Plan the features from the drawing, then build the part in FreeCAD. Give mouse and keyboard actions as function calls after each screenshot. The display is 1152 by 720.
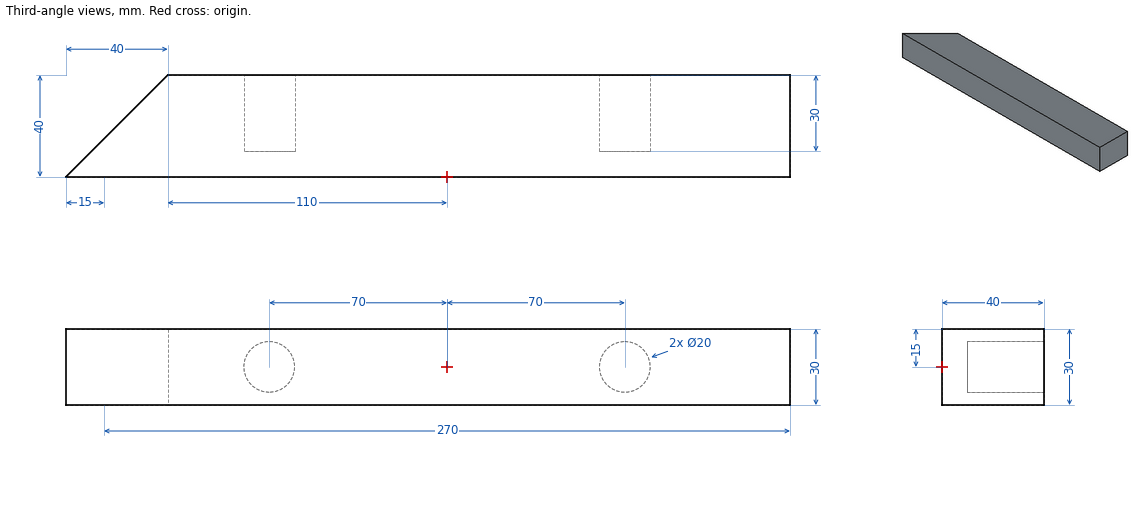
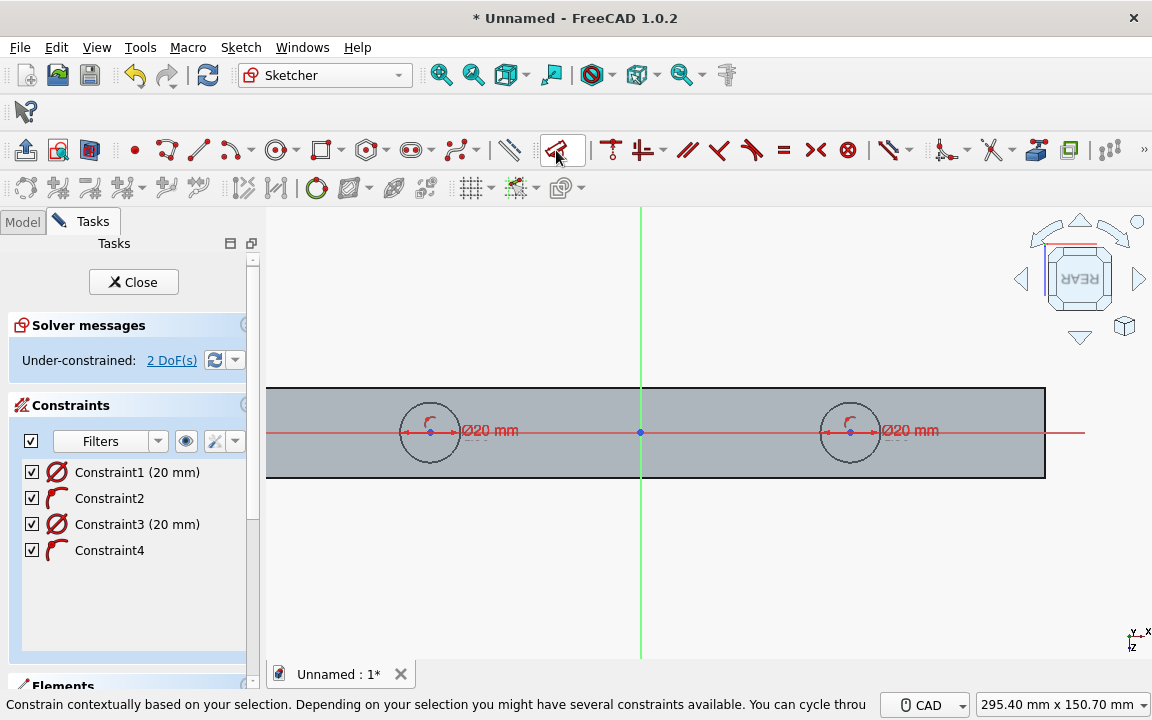
click(850, 433)
click(745, 467)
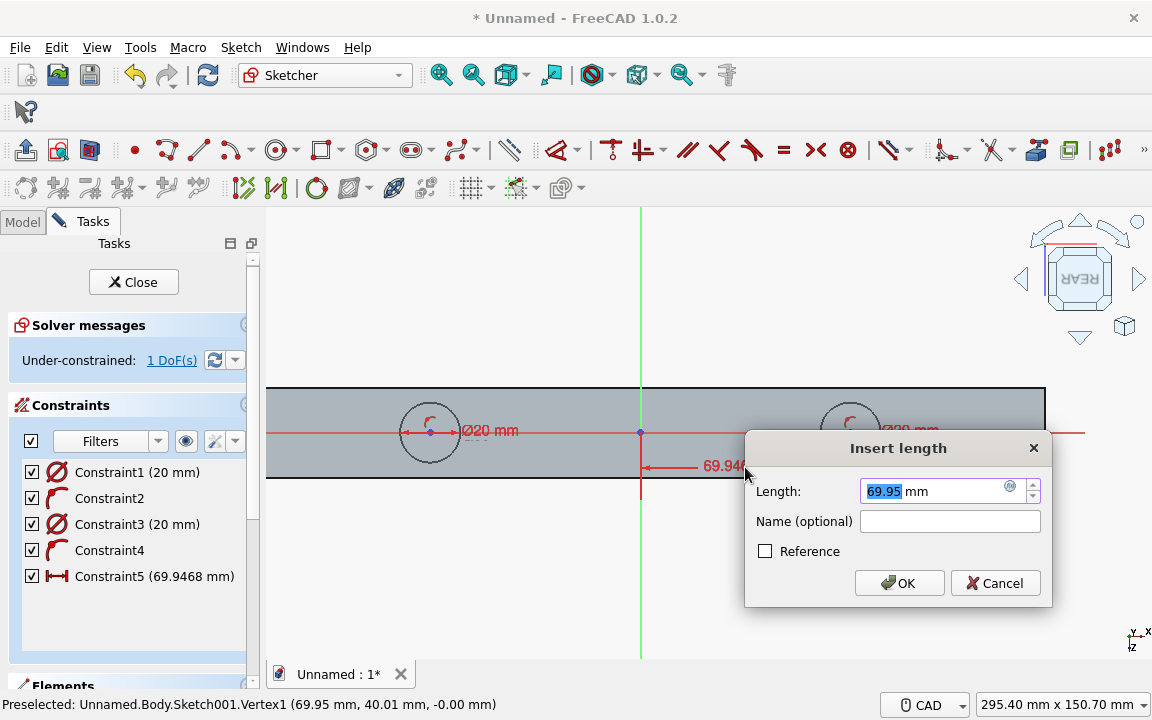
text(70)
key(Return)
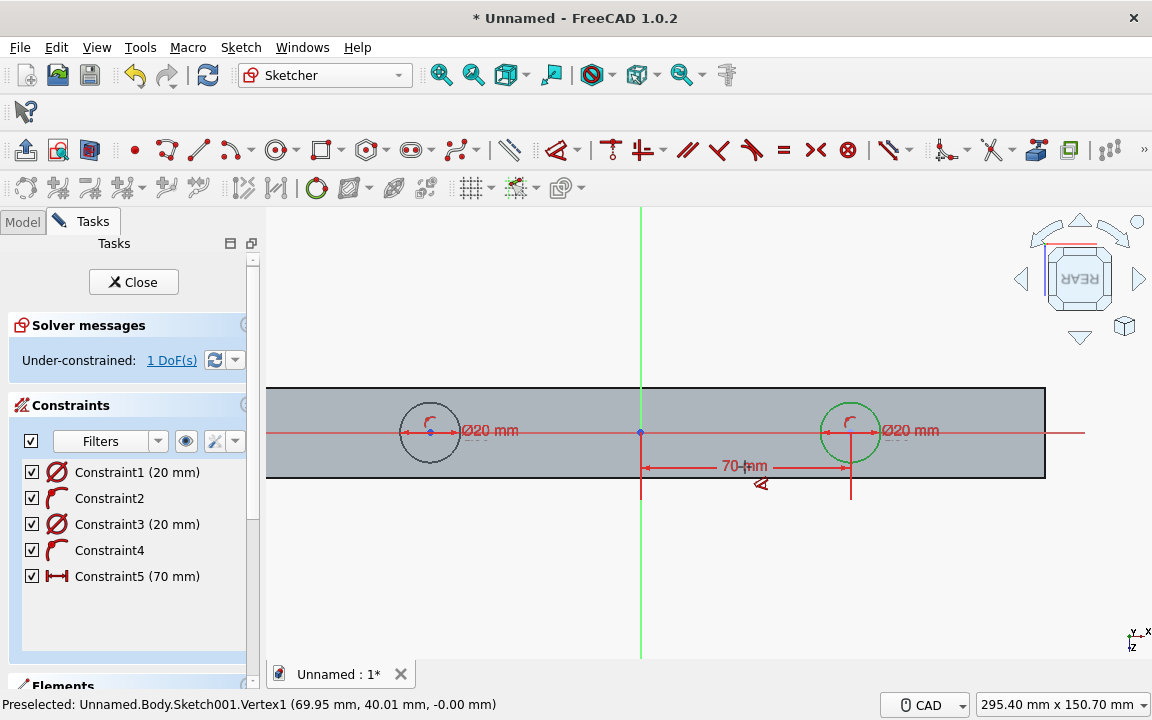
click(430, 433)
click(535, 467)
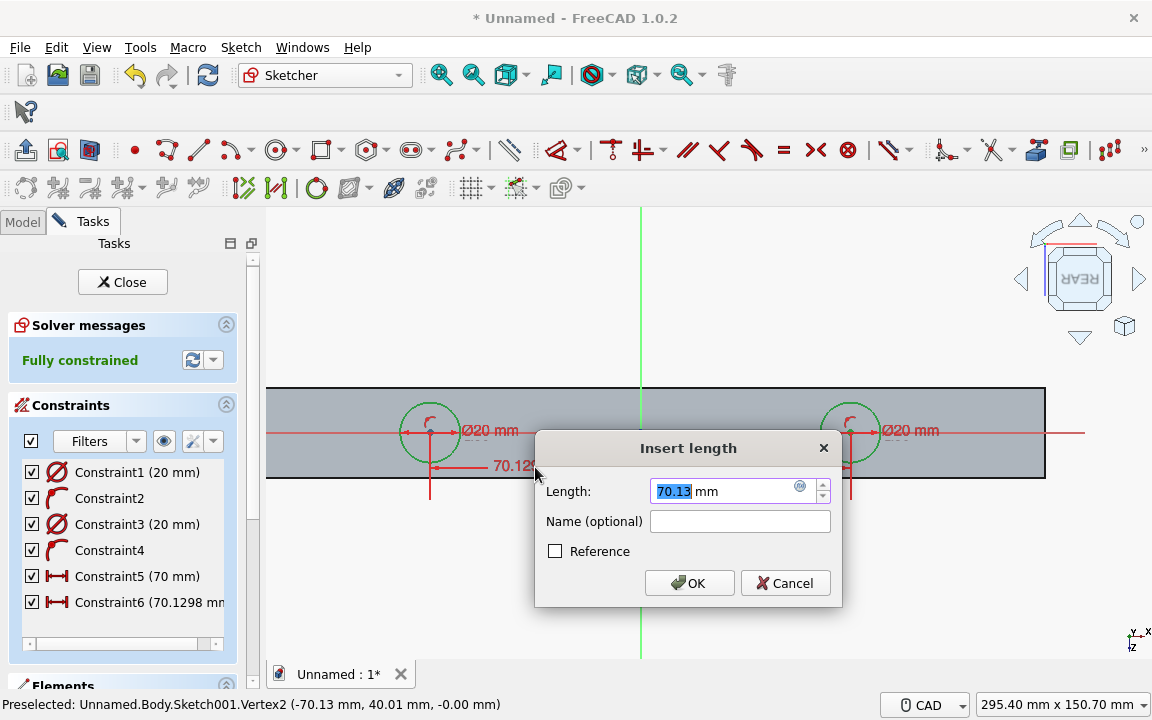
text(70)
key(Return)
key(Escape)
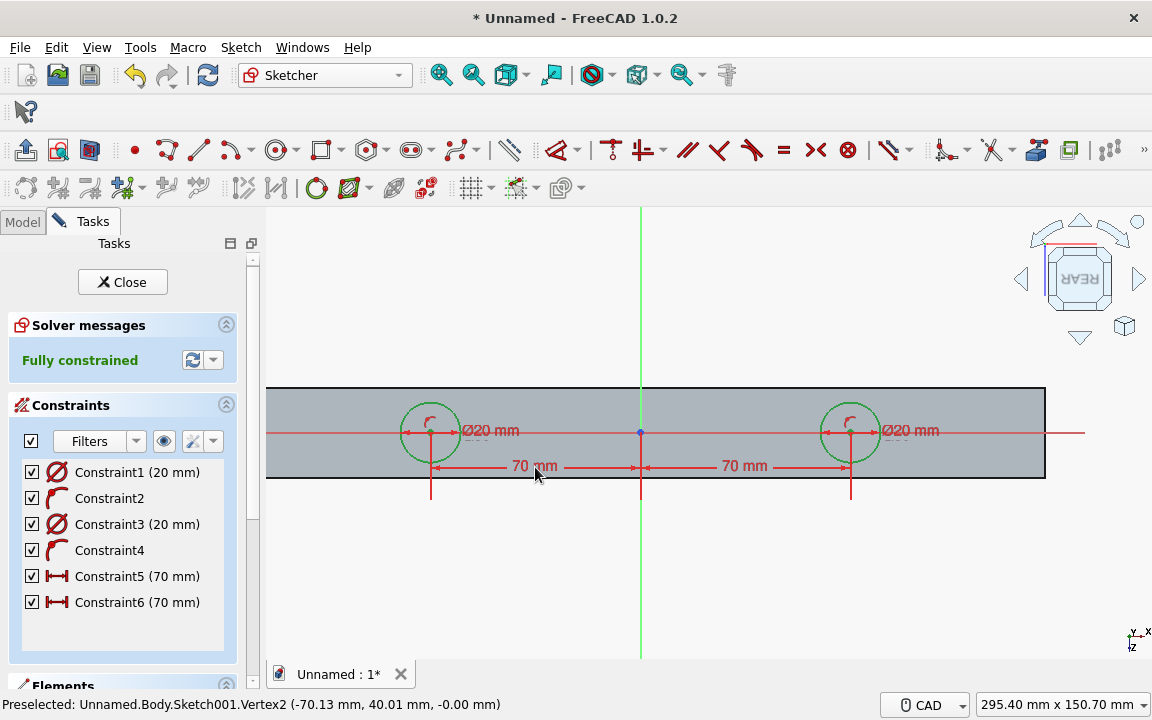
click(123, 282)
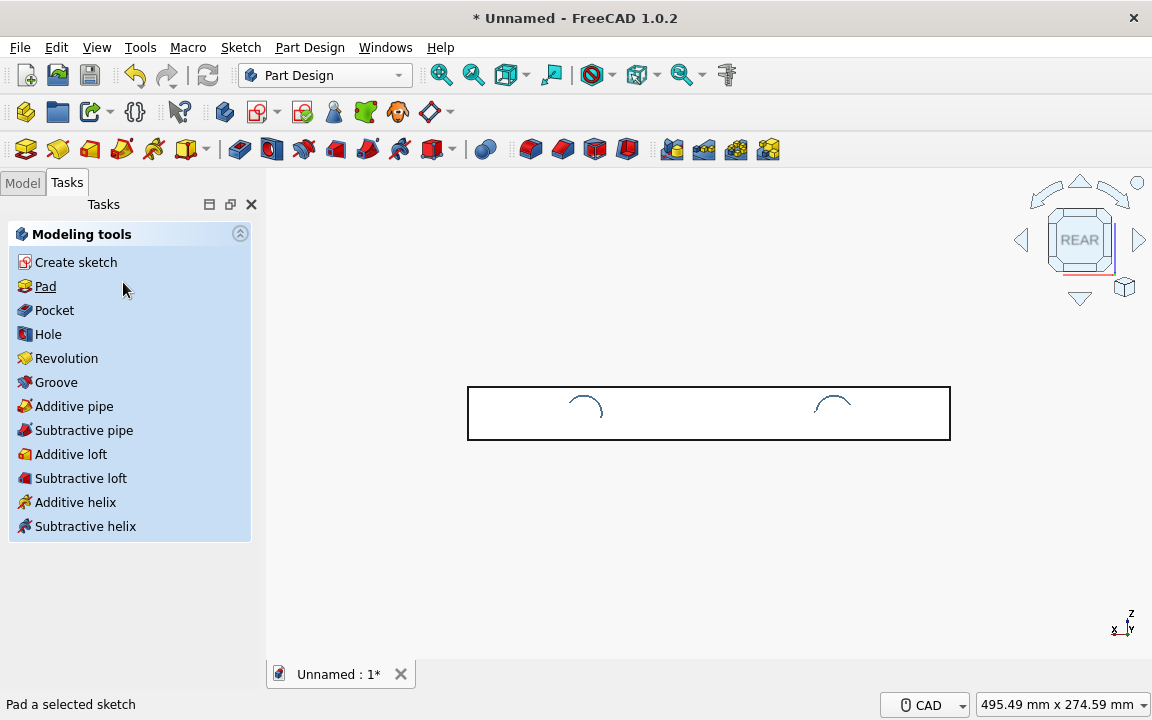
click(240, 150)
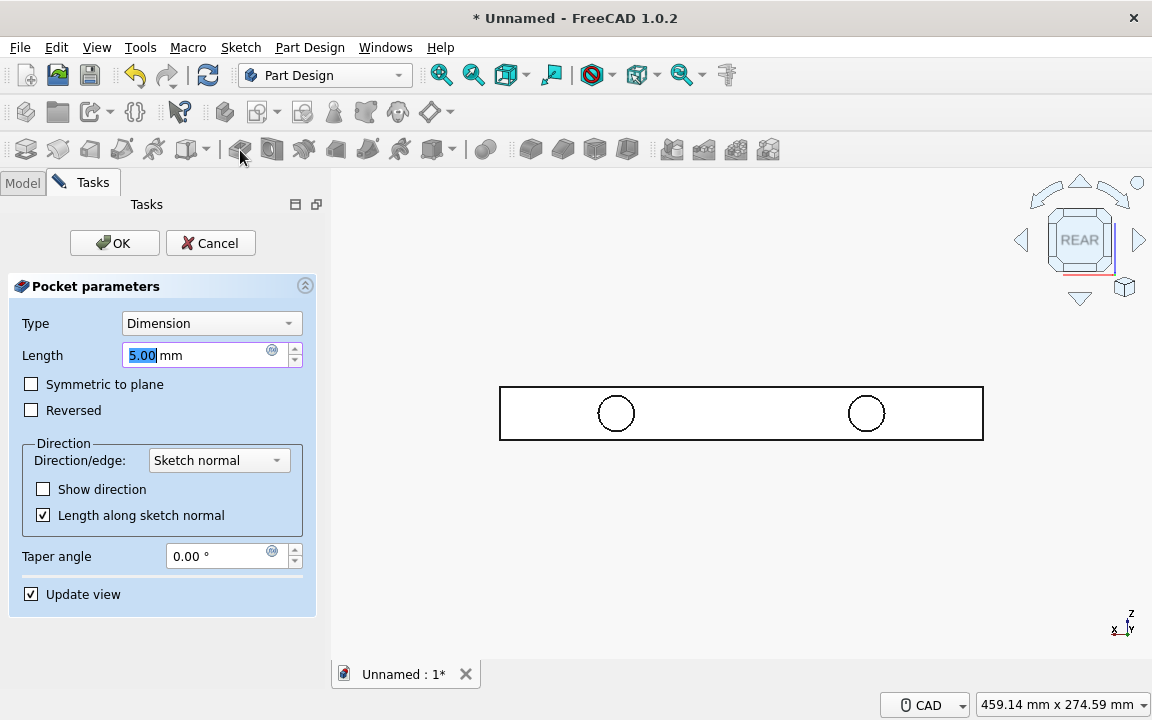
text(30)
key(Tab)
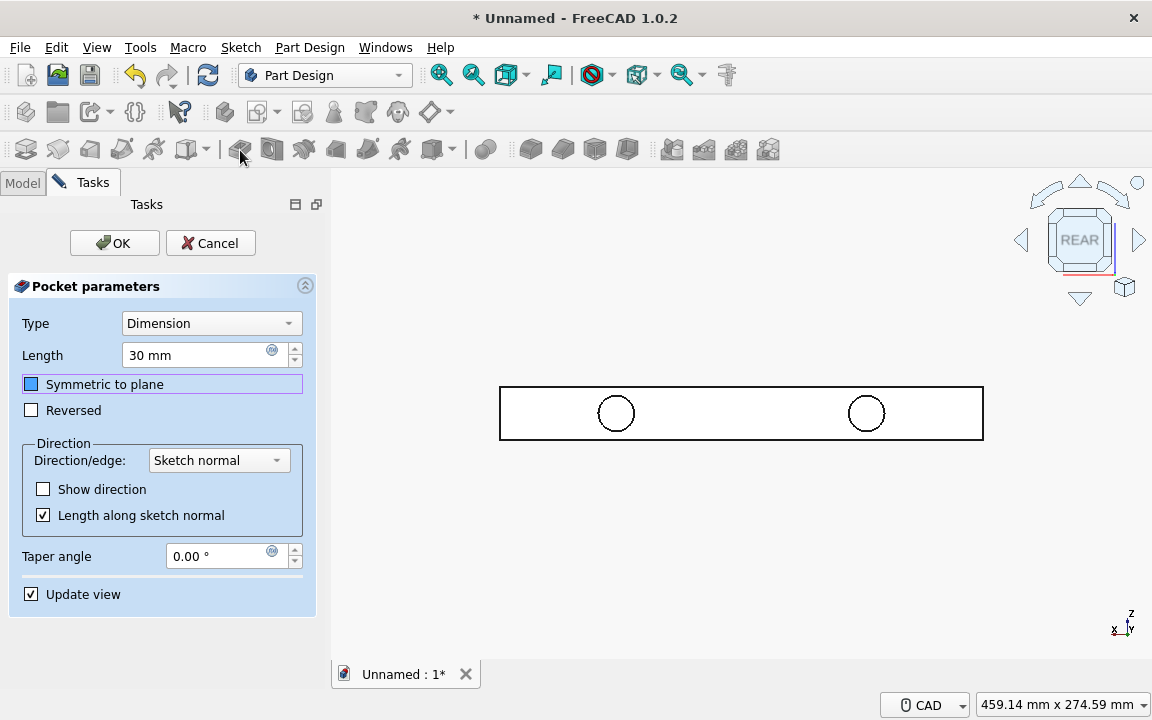
click(115, 243)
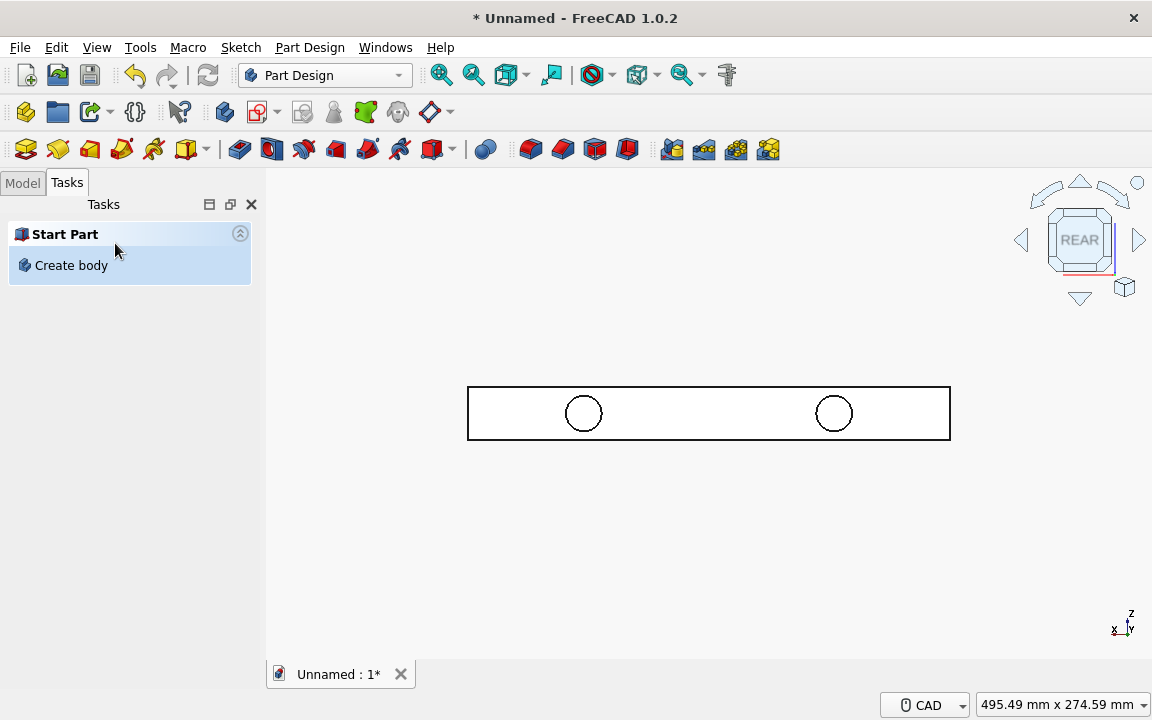
key(6)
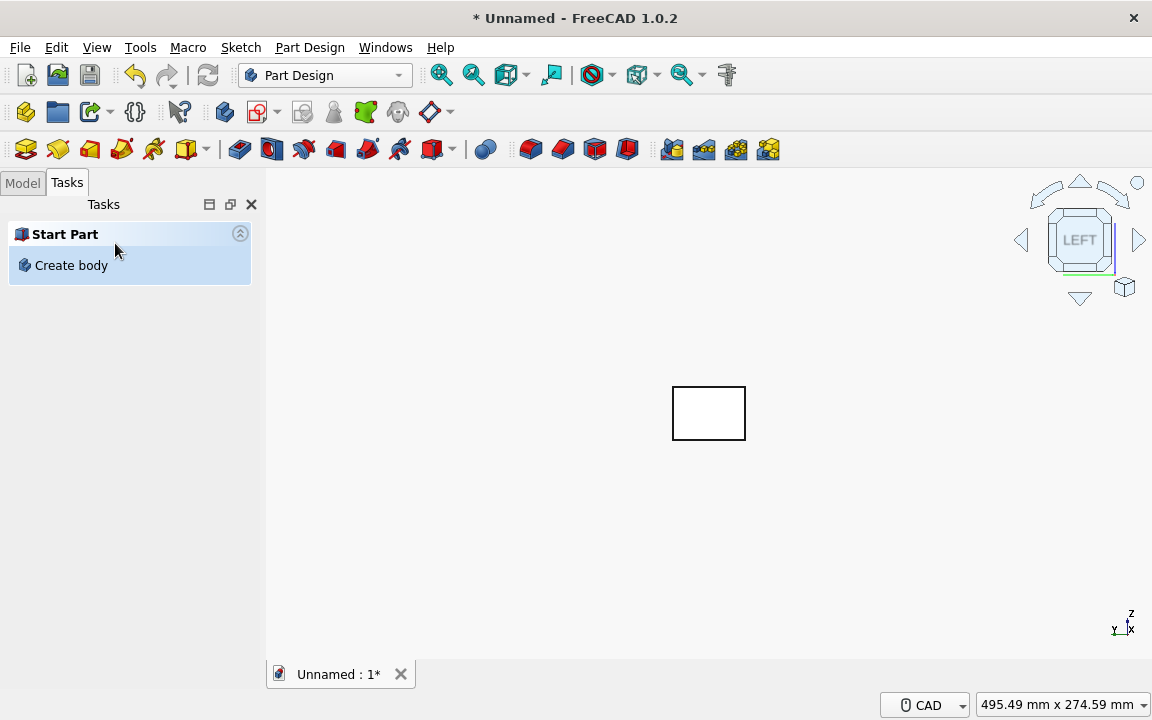
click(442, 76)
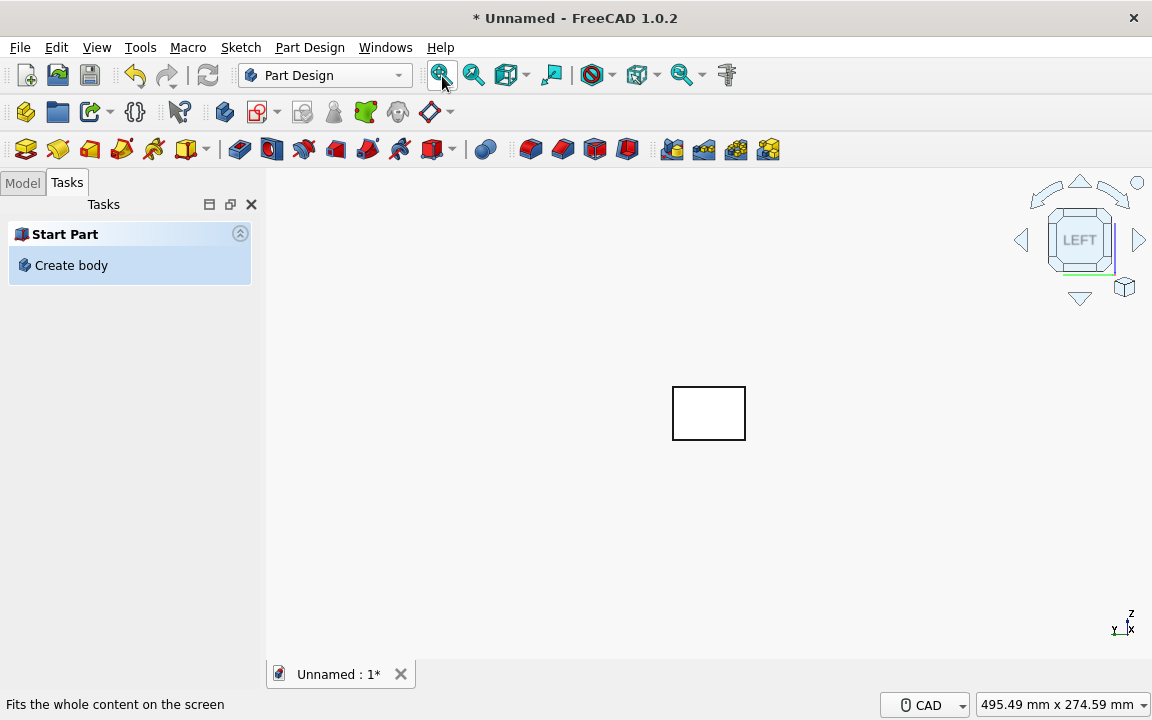
click(709, 412)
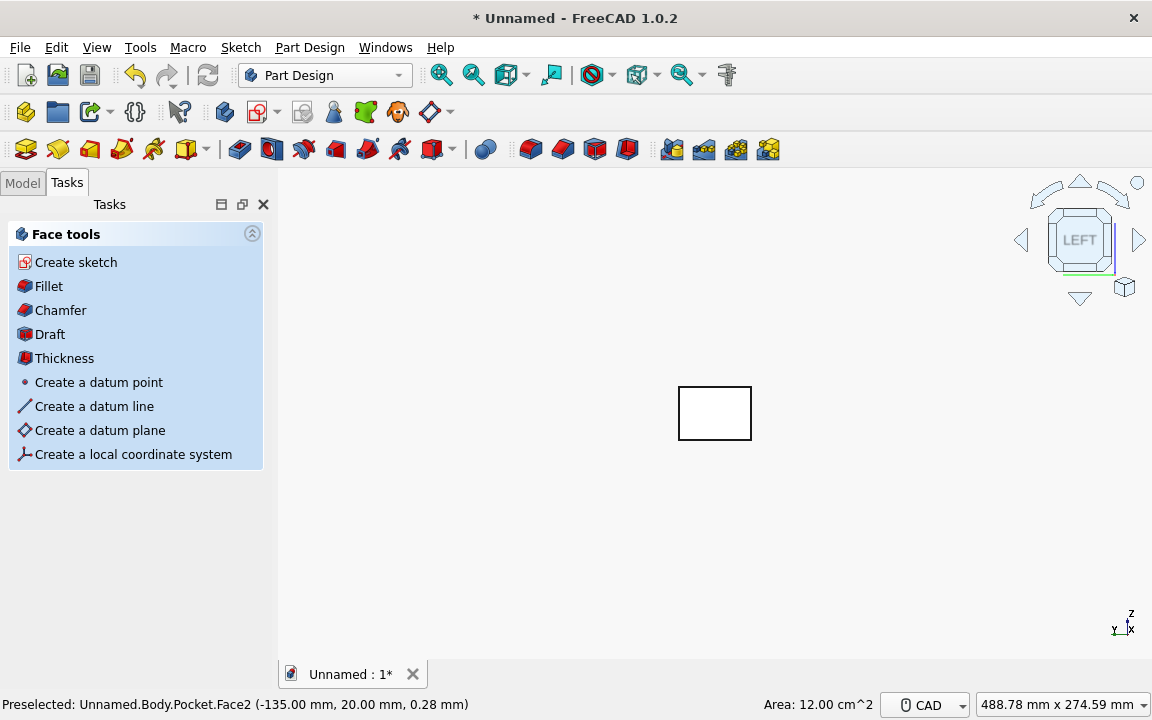
click(258, 112)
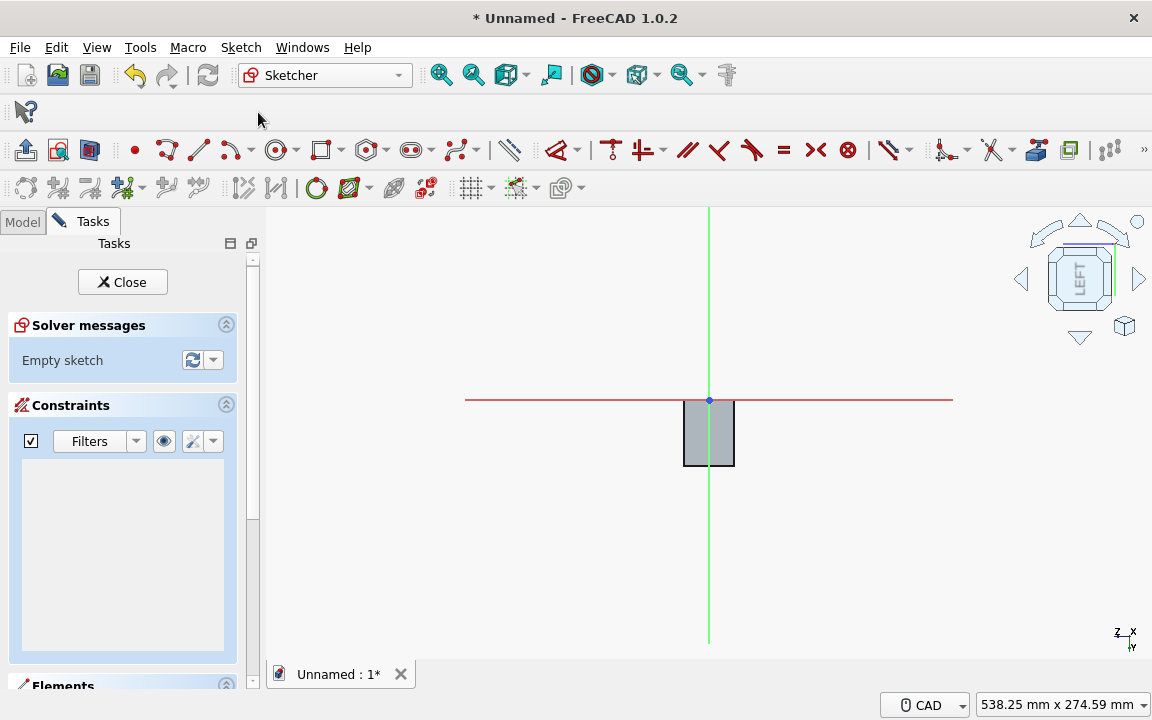
scroll(731, 433, up, 7)